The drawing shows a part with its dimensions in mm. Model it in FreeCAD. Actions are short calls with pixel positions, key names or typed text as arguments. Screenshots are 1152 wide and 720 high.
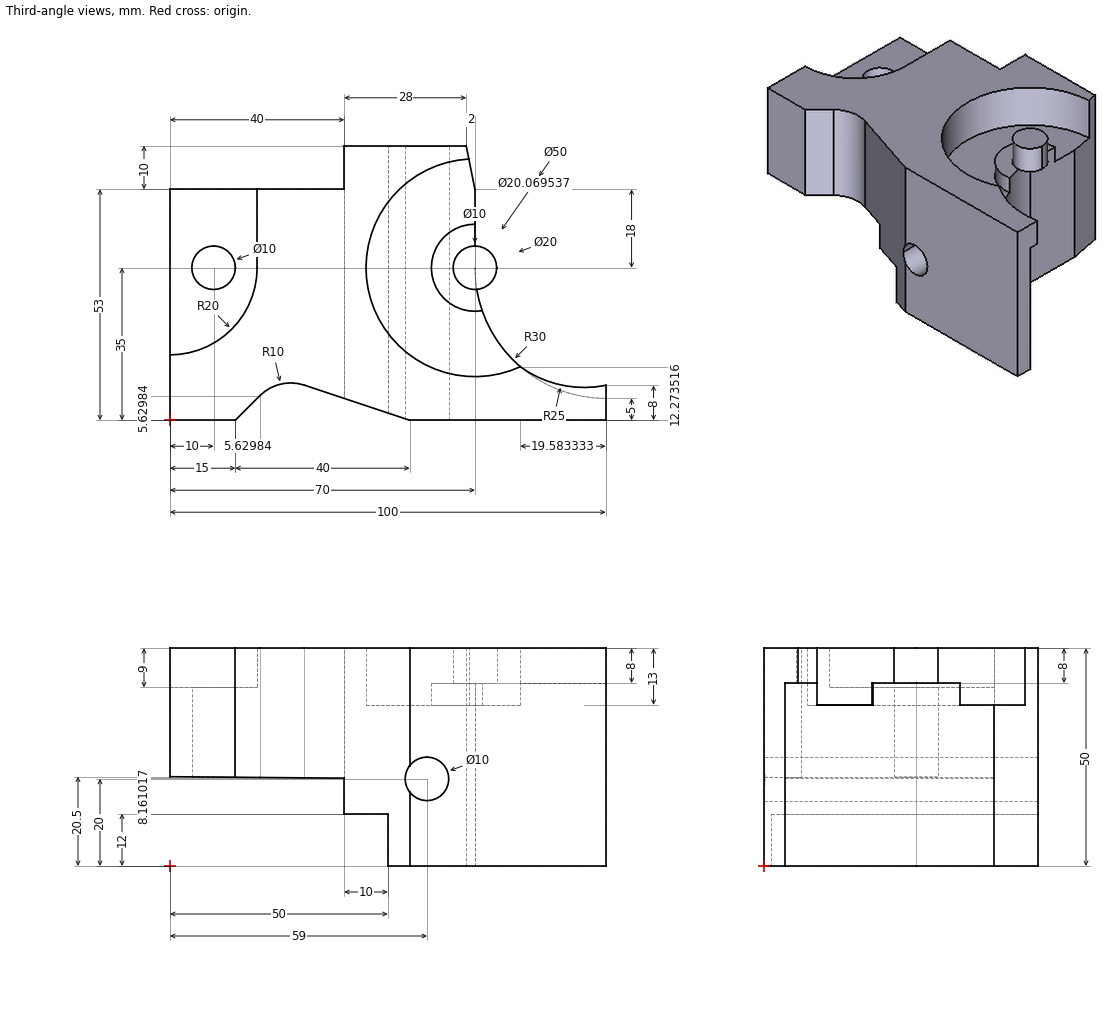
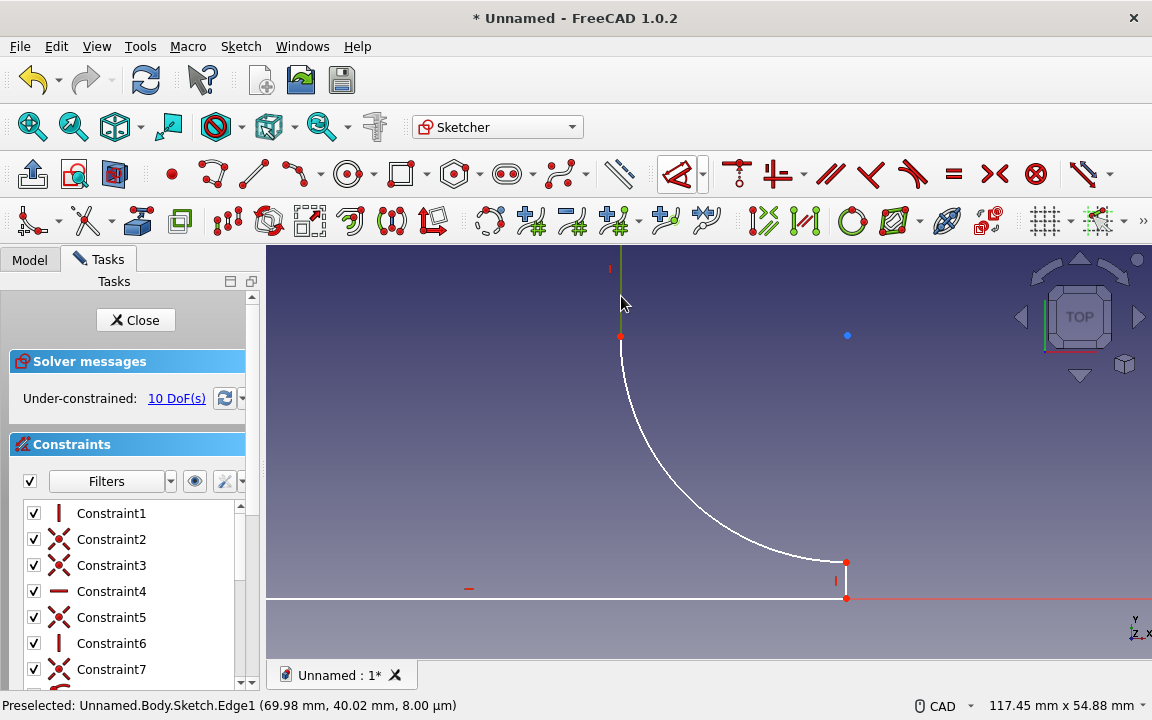
click(645, 439)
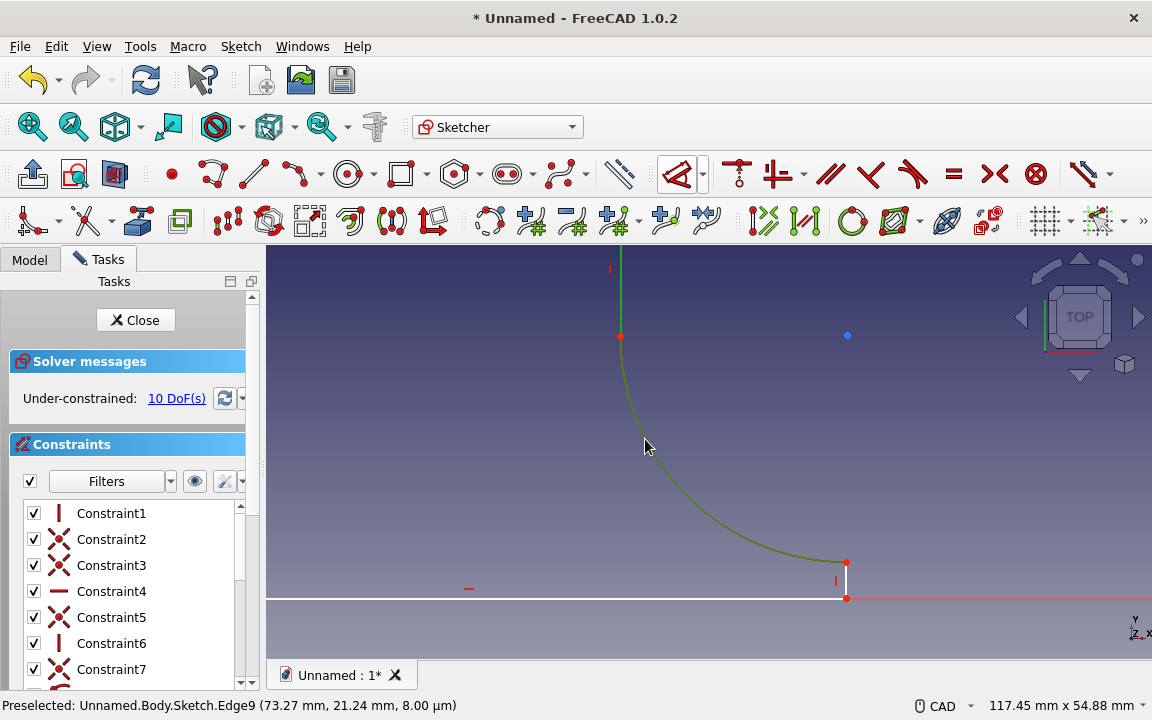
key(t)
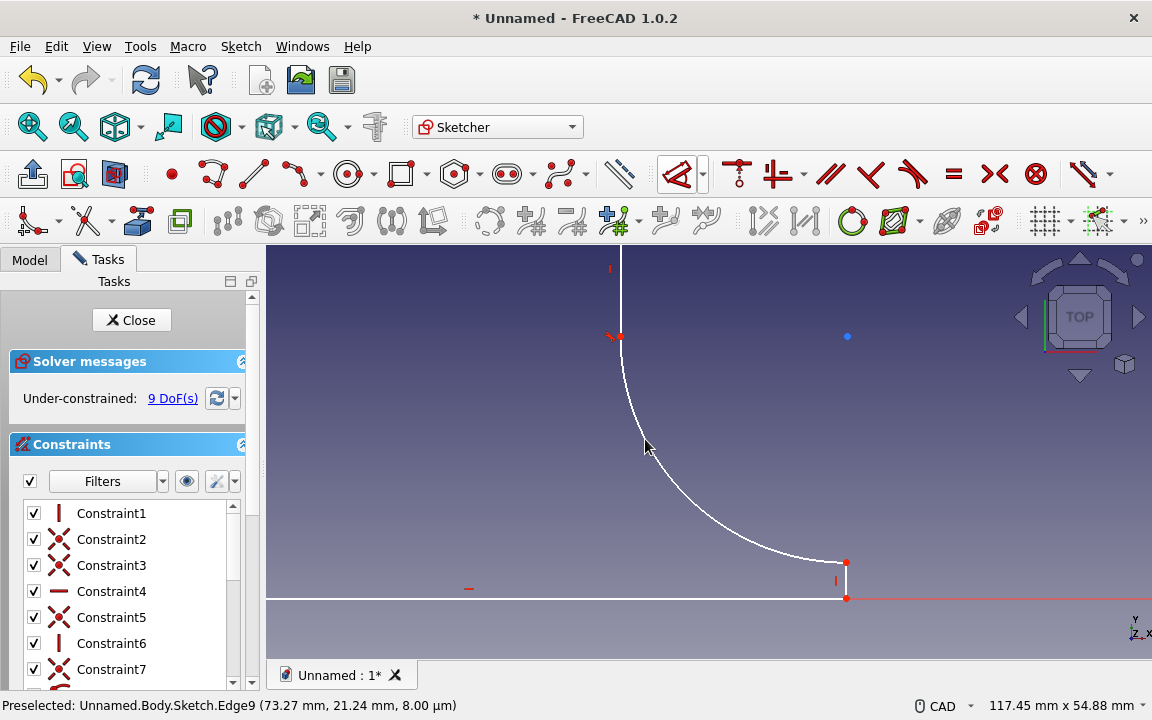
click(676, 174)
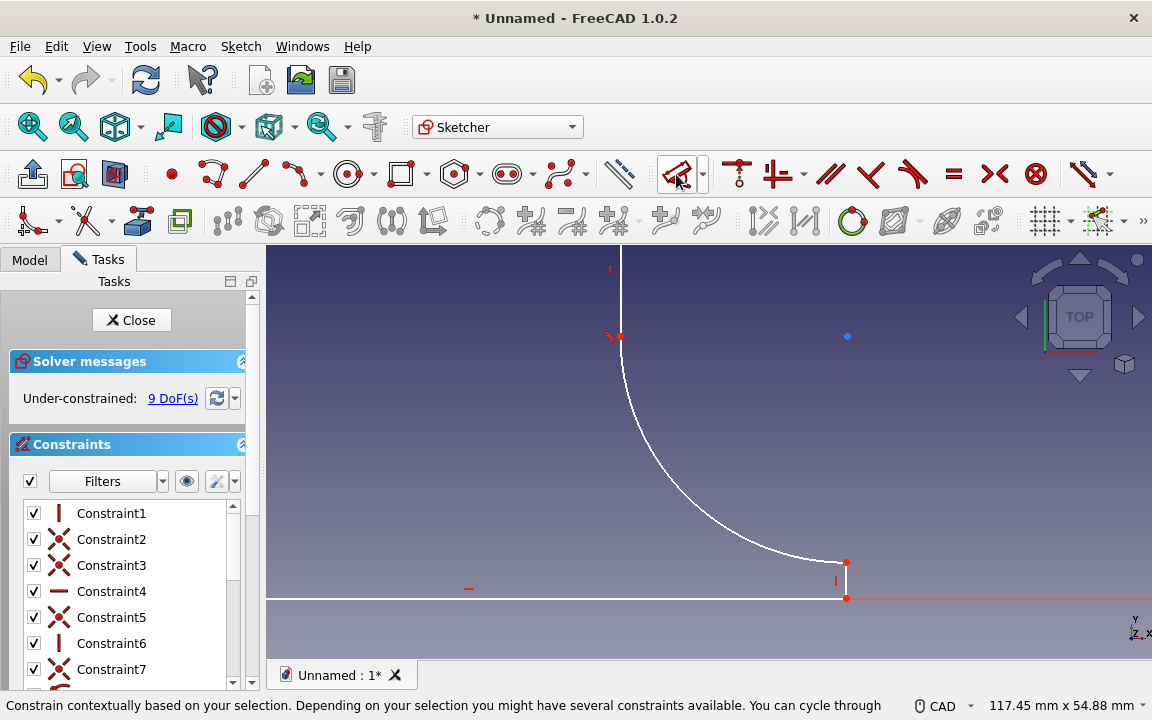
click(645, 439)
click(616, 454)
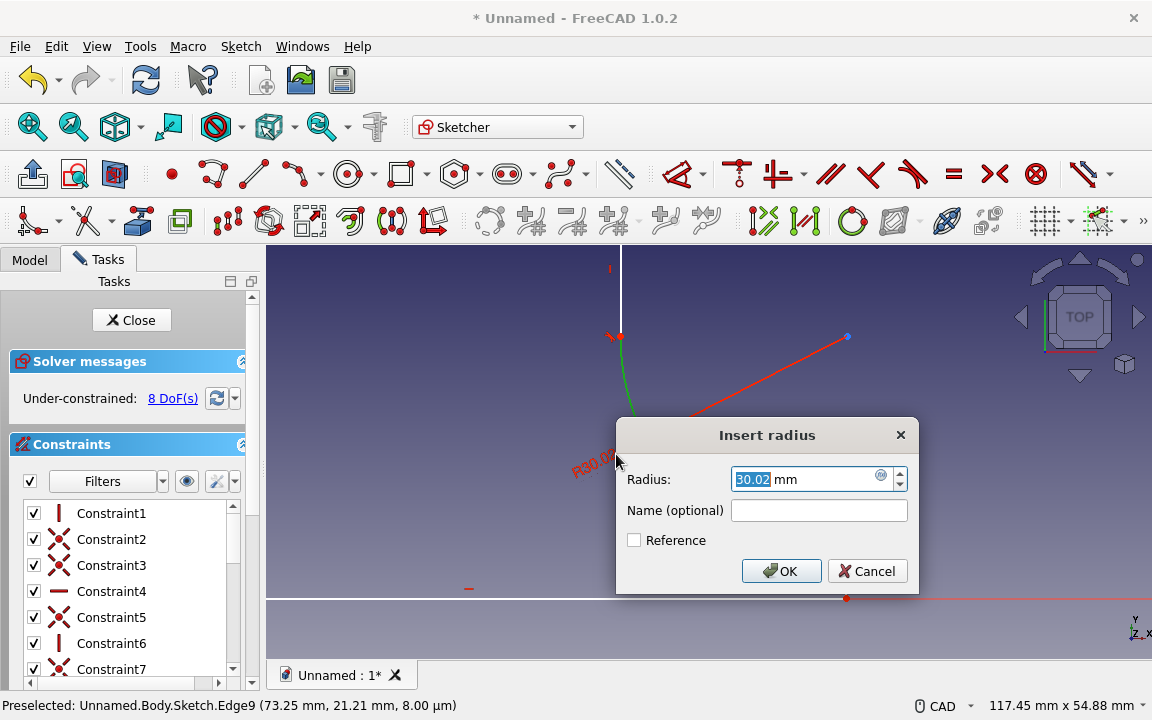
text(30)
key(Return)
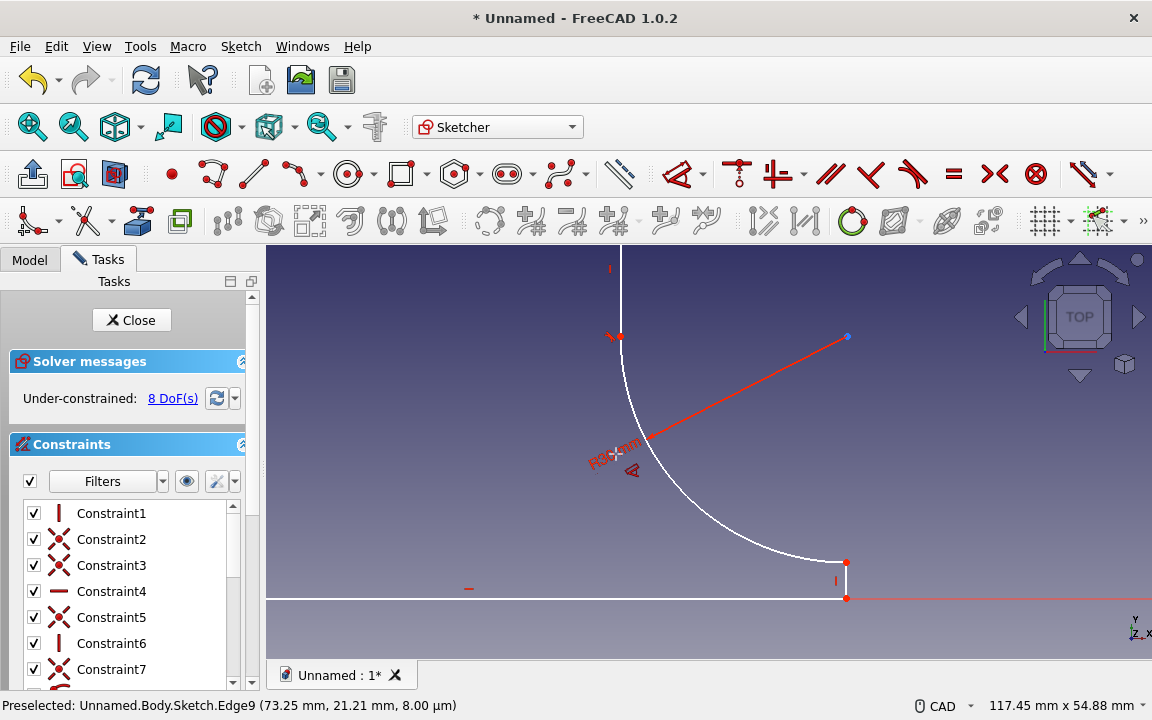
scroll(846, 588, up, 2)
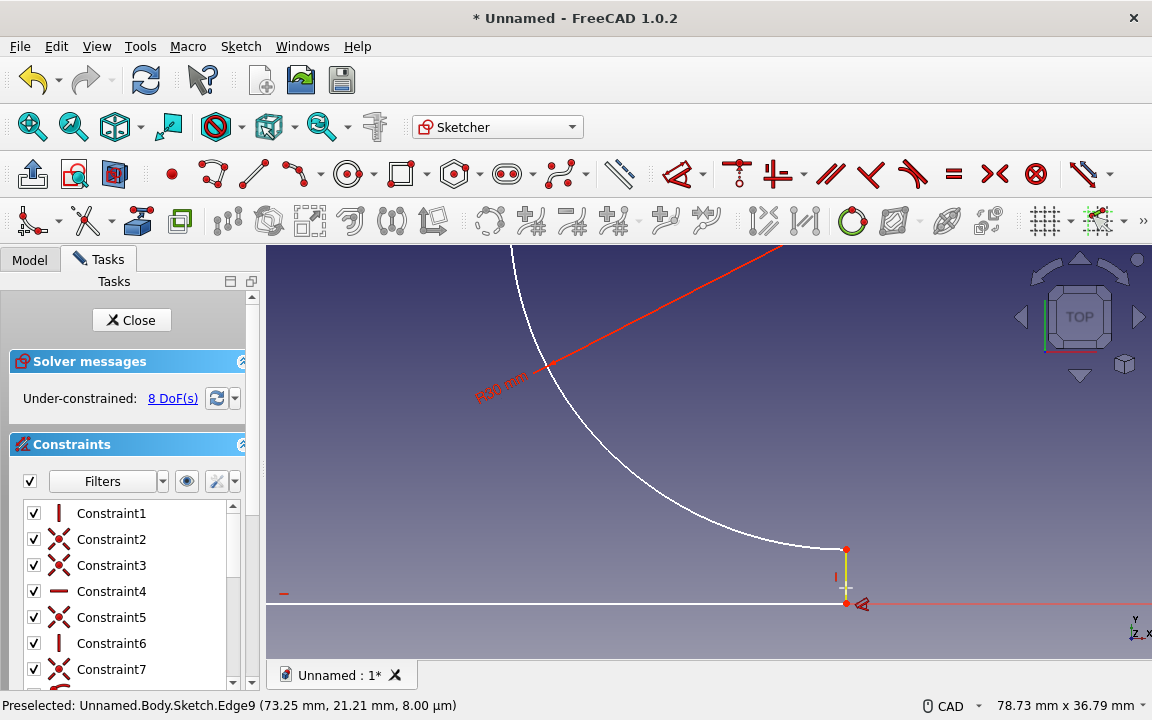
click(846, 588)
click(880, 577)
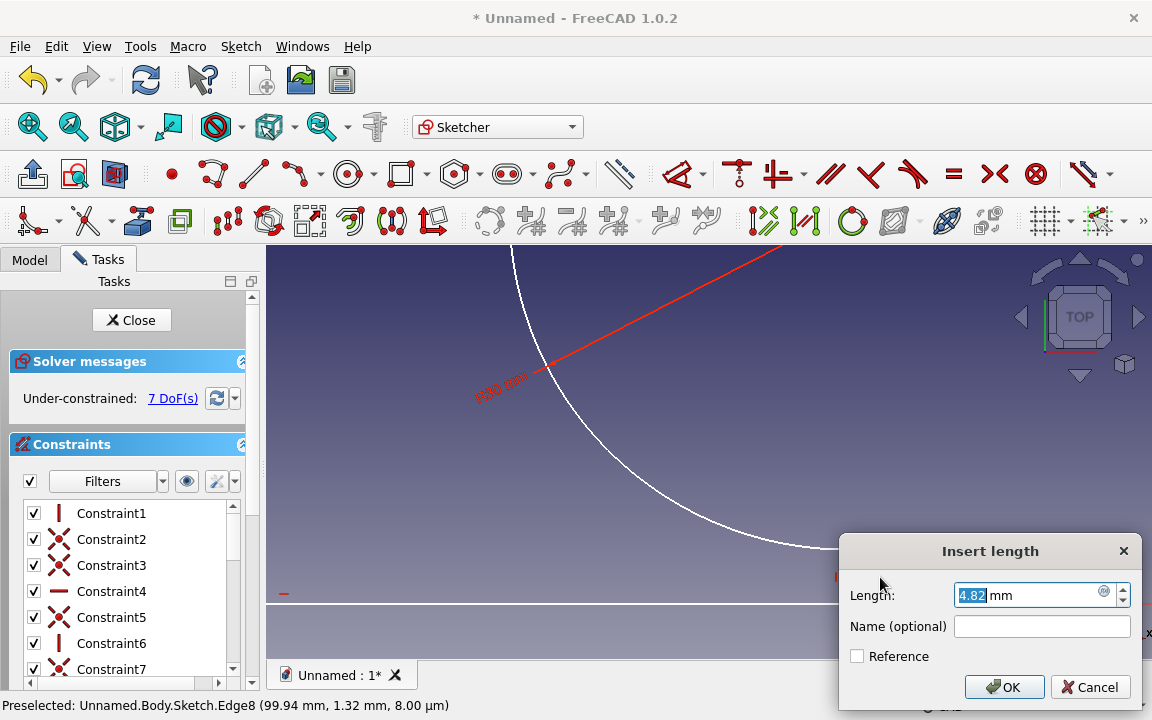
text(5)
key(Return)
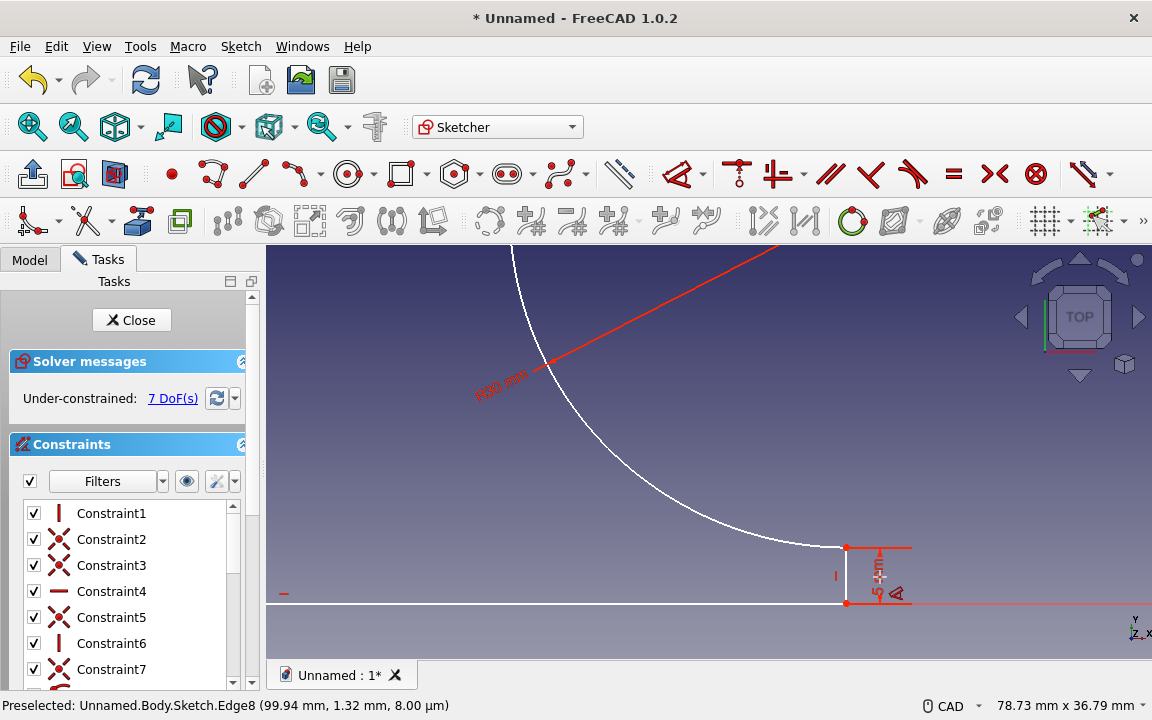
scroll(848, 570, down, 5)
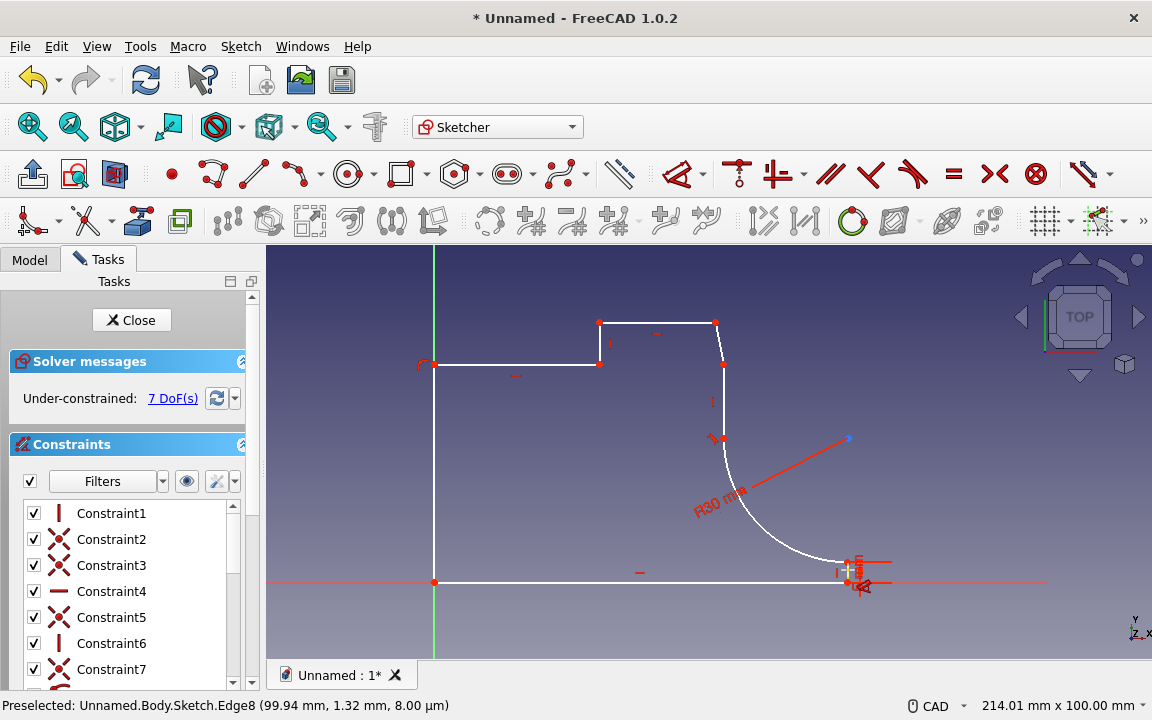
click(724, 416)
click(758, 401)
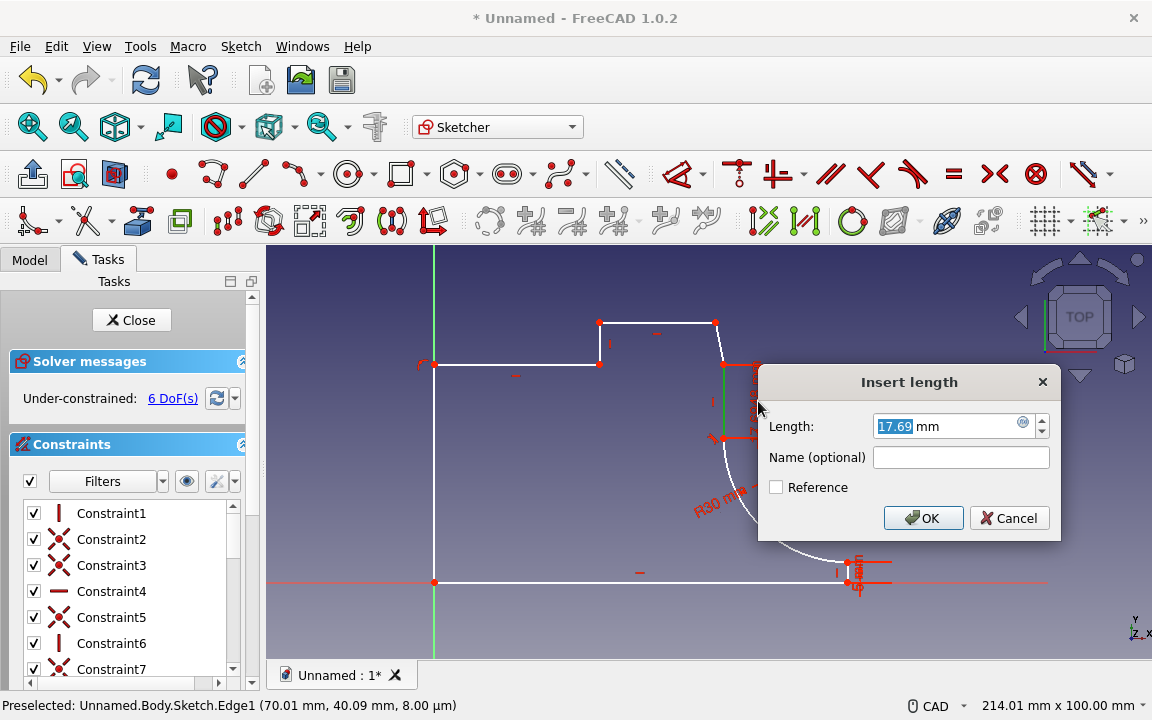
text(18)
key(Return)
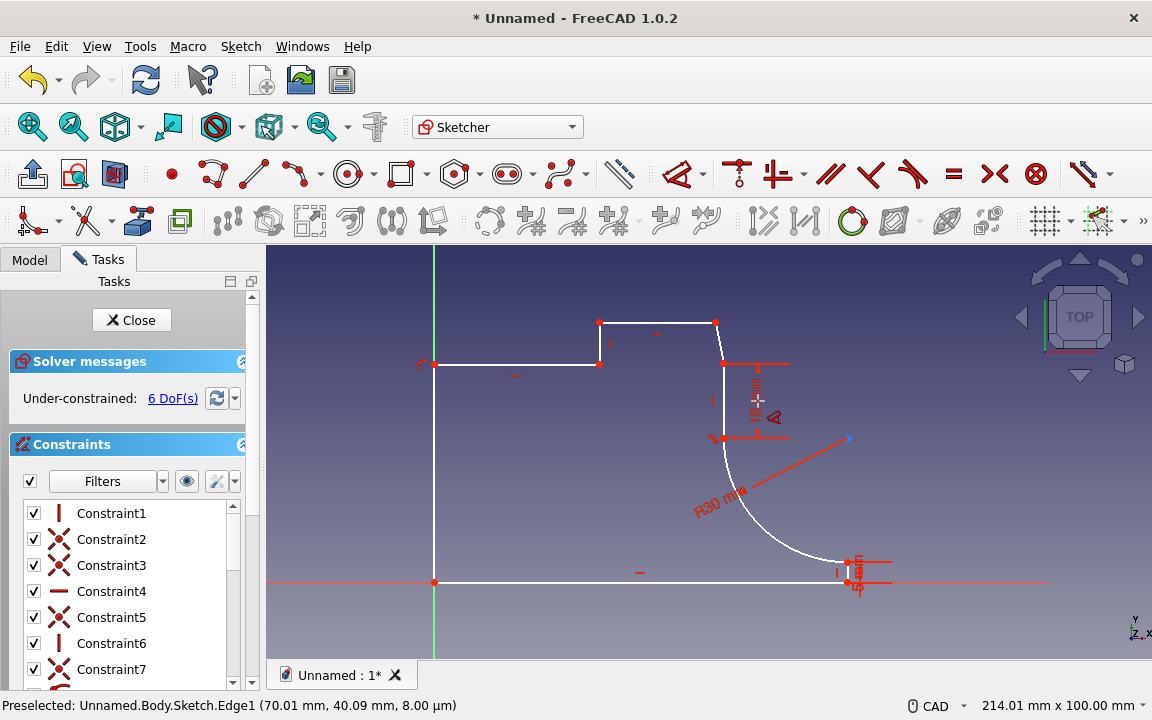
click(681, 323)
click(658, 289)